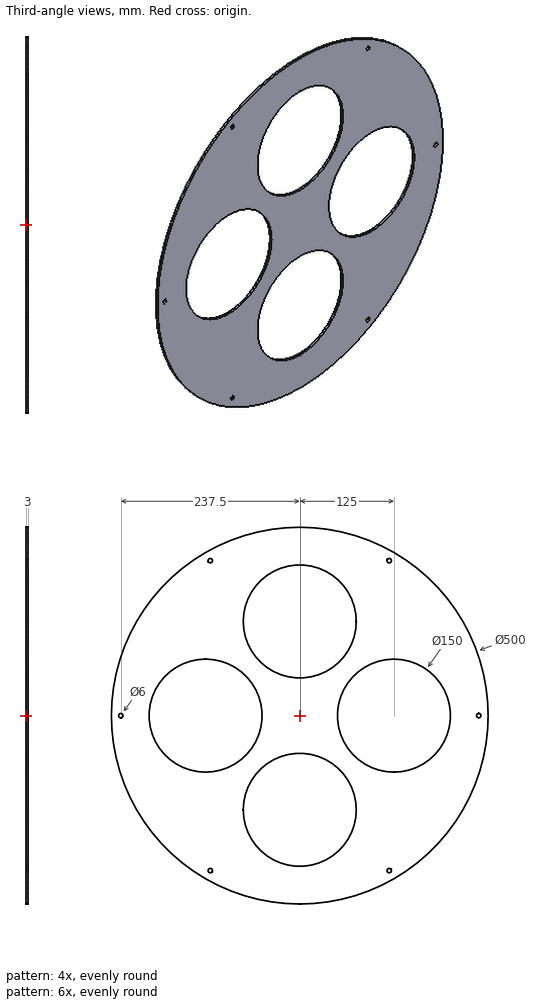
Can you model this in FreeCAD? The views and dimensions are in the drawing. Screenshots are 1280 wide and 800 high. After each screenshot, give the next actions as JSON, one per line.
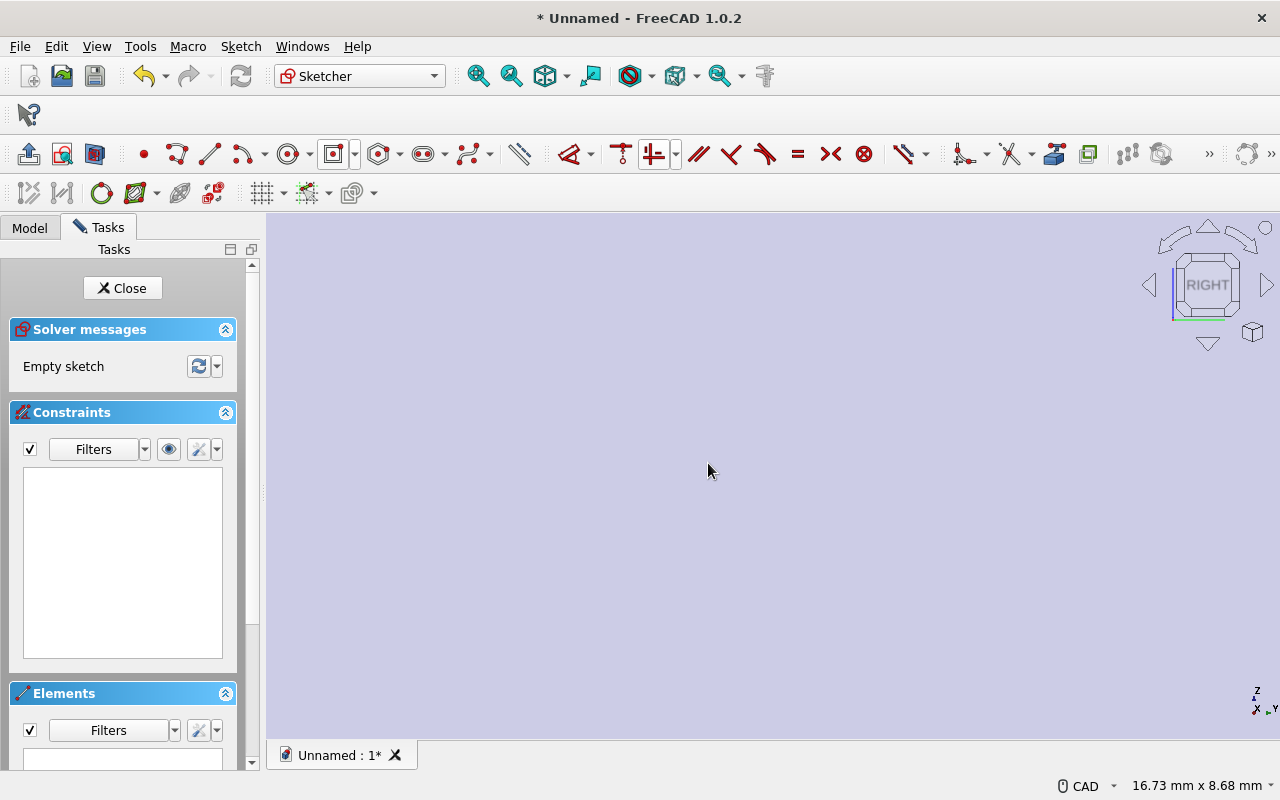
{"action": "left_click", "coordinate": [288, 154]}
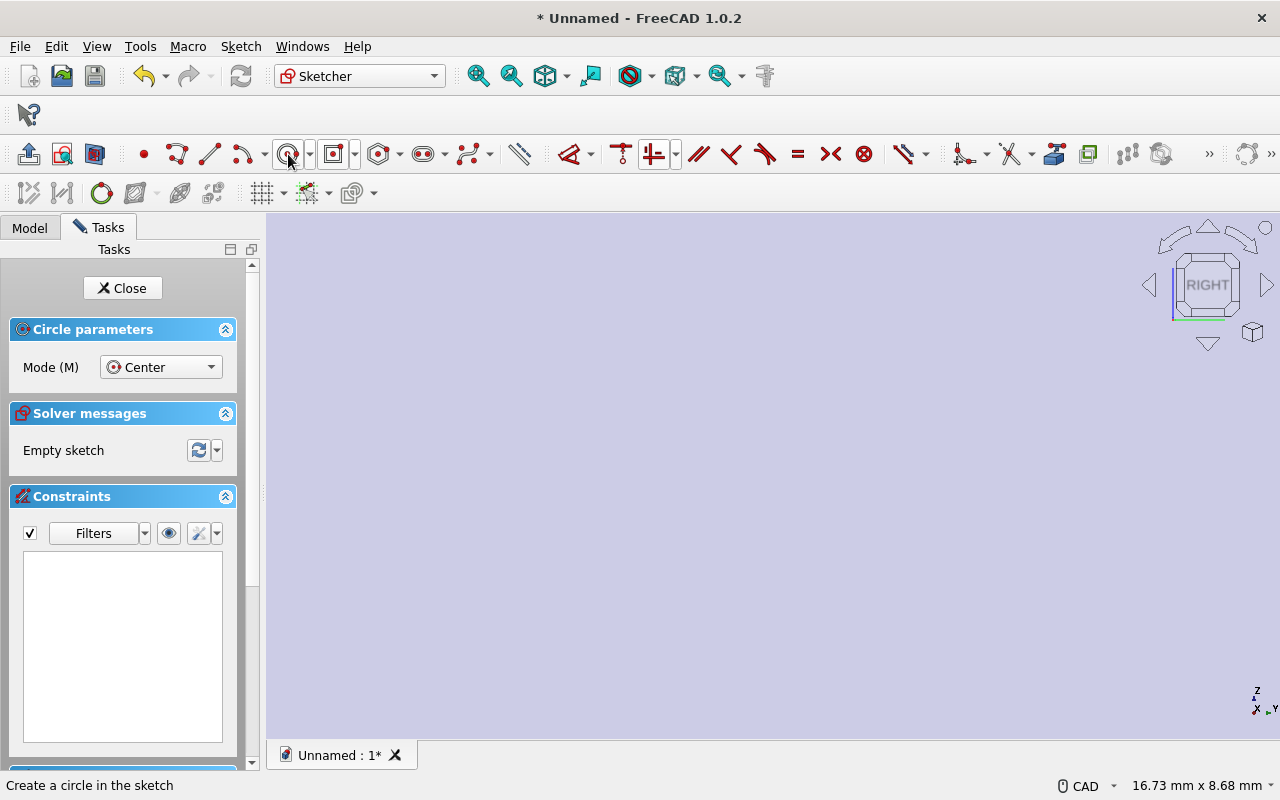
{"action": "left_click", "coordinate": [702, 475]}
{"action": "mouse_move", "coordinate": [830, 347]}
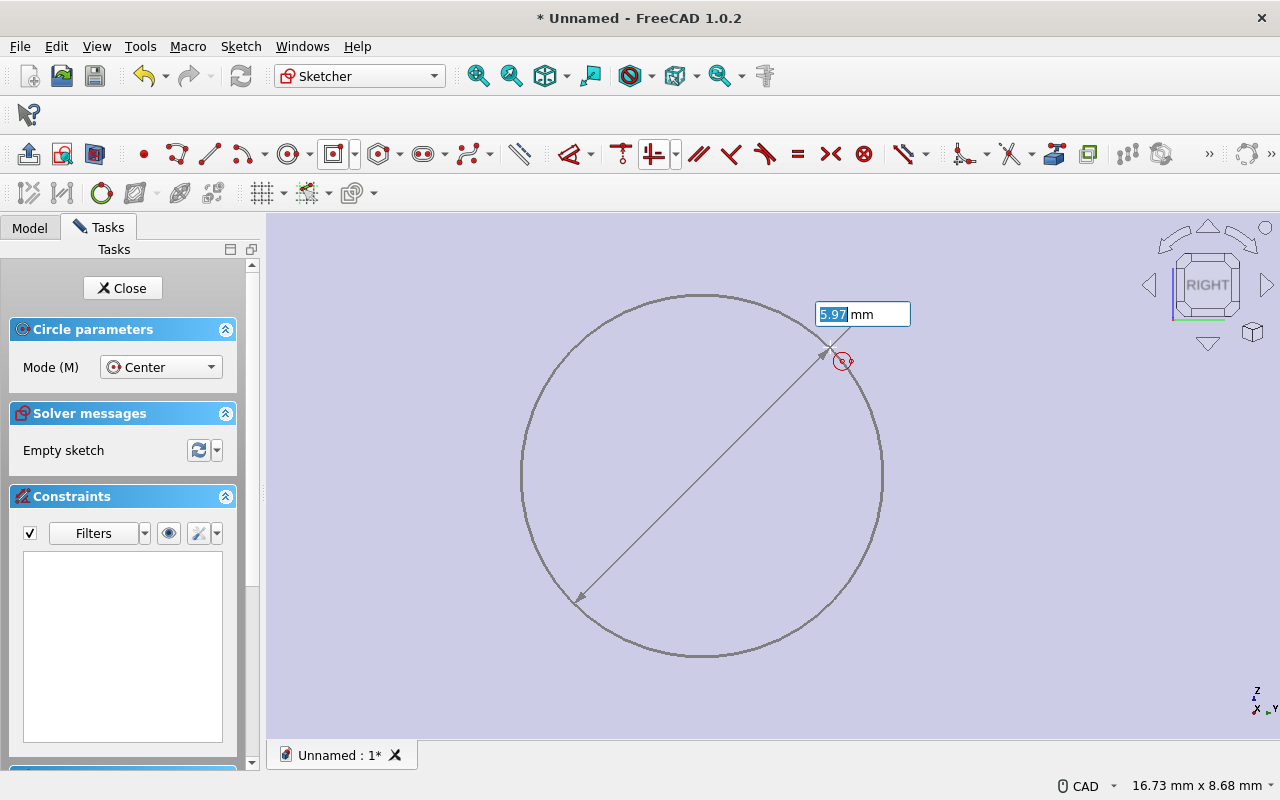
{"action": "type", "text": "6"}
{"action": "key", "text": "Return"}
{"action": "key", "text": "Escape"}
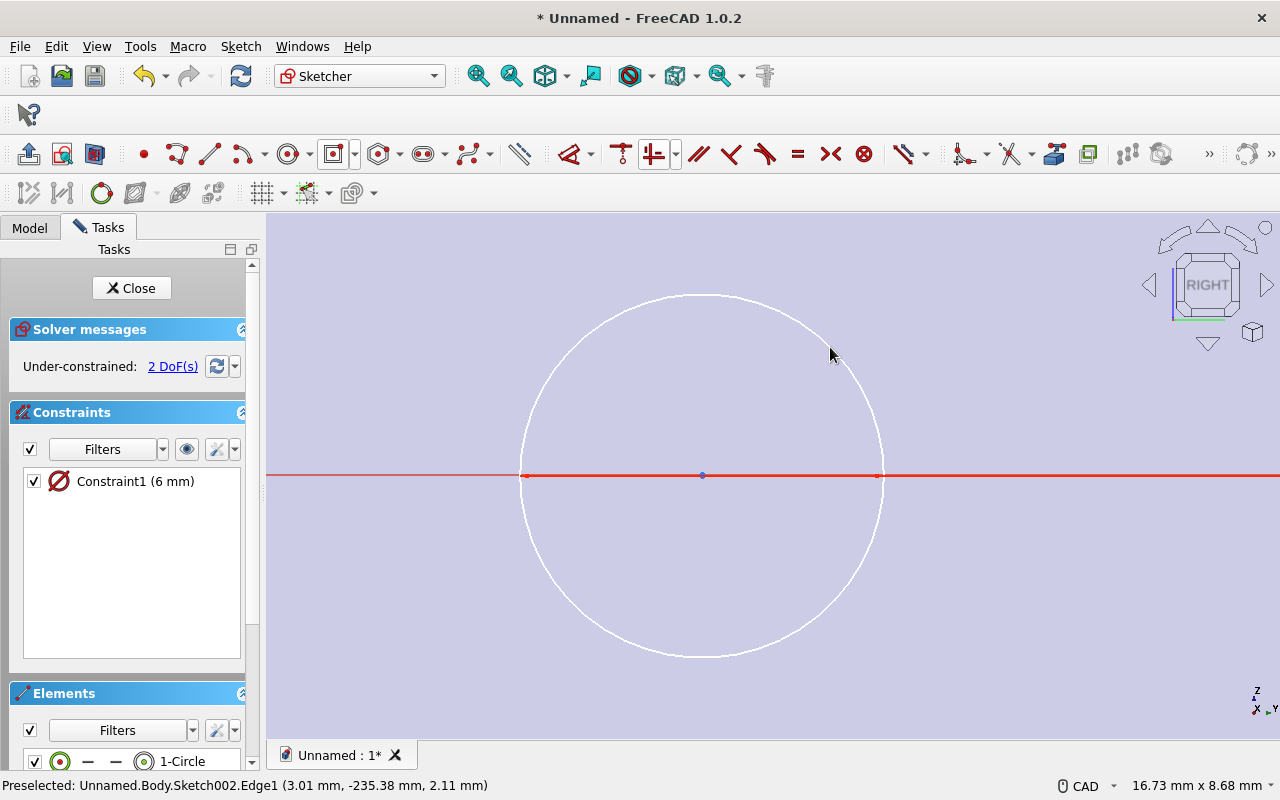
{"action": "left_click", "coordinate": [702, 476]}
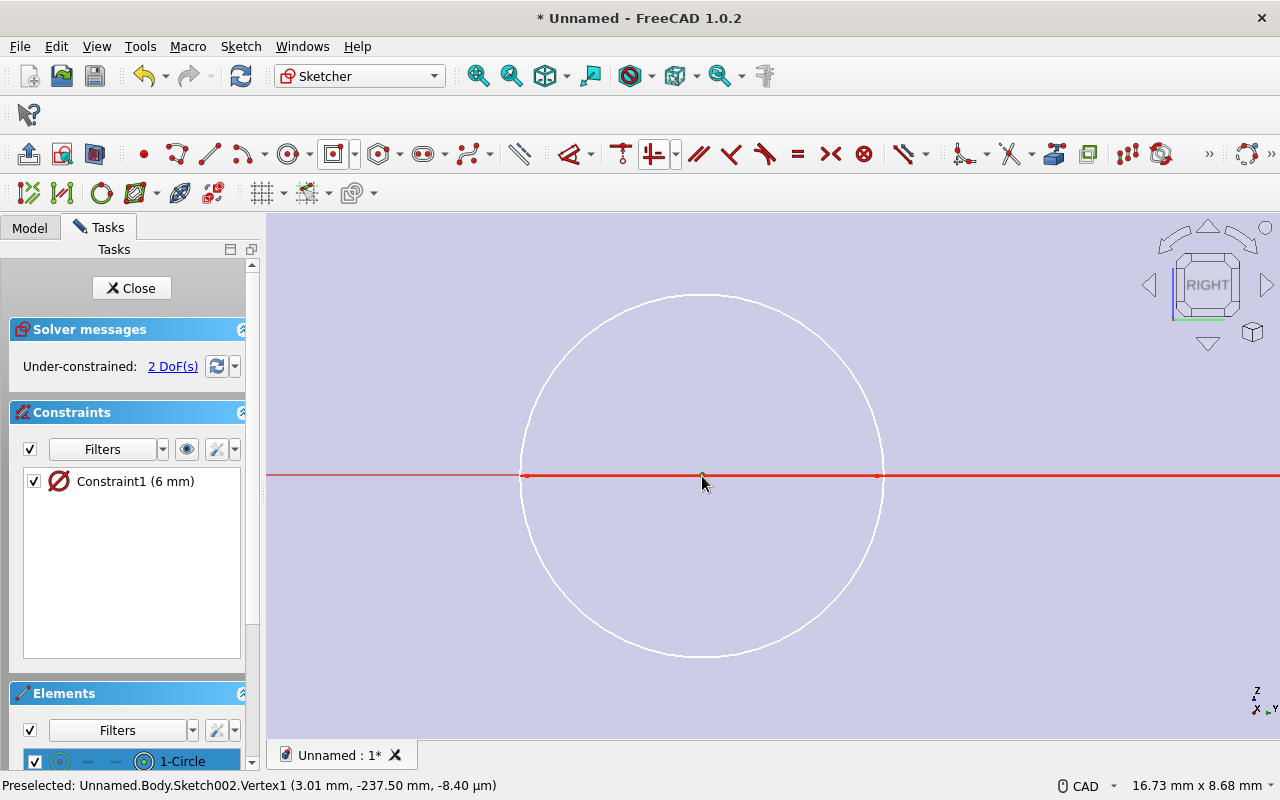
{"action": "left_click", "coordinate": [353, 475]}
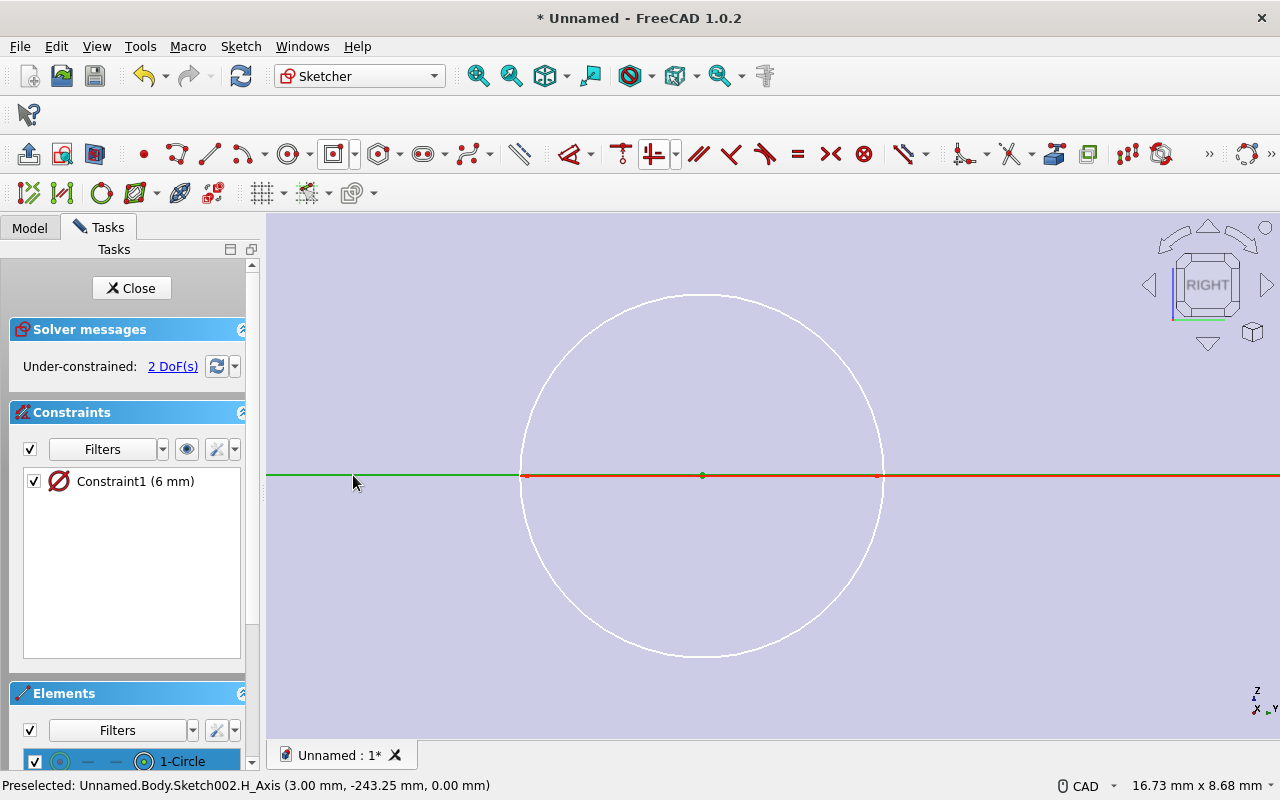
{"action": "left_click", "coordinate": [621, 154]}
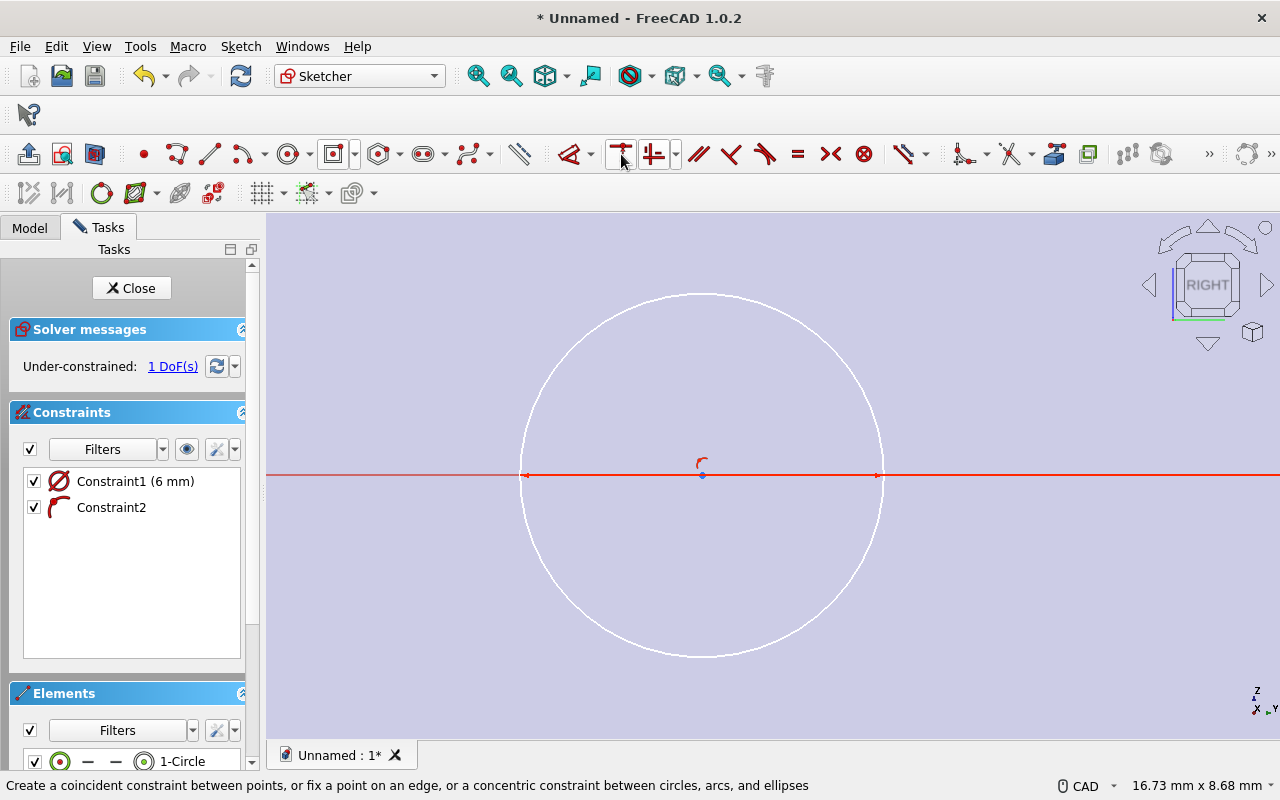
{"action": "left_click", "coordinate": [568, 154]}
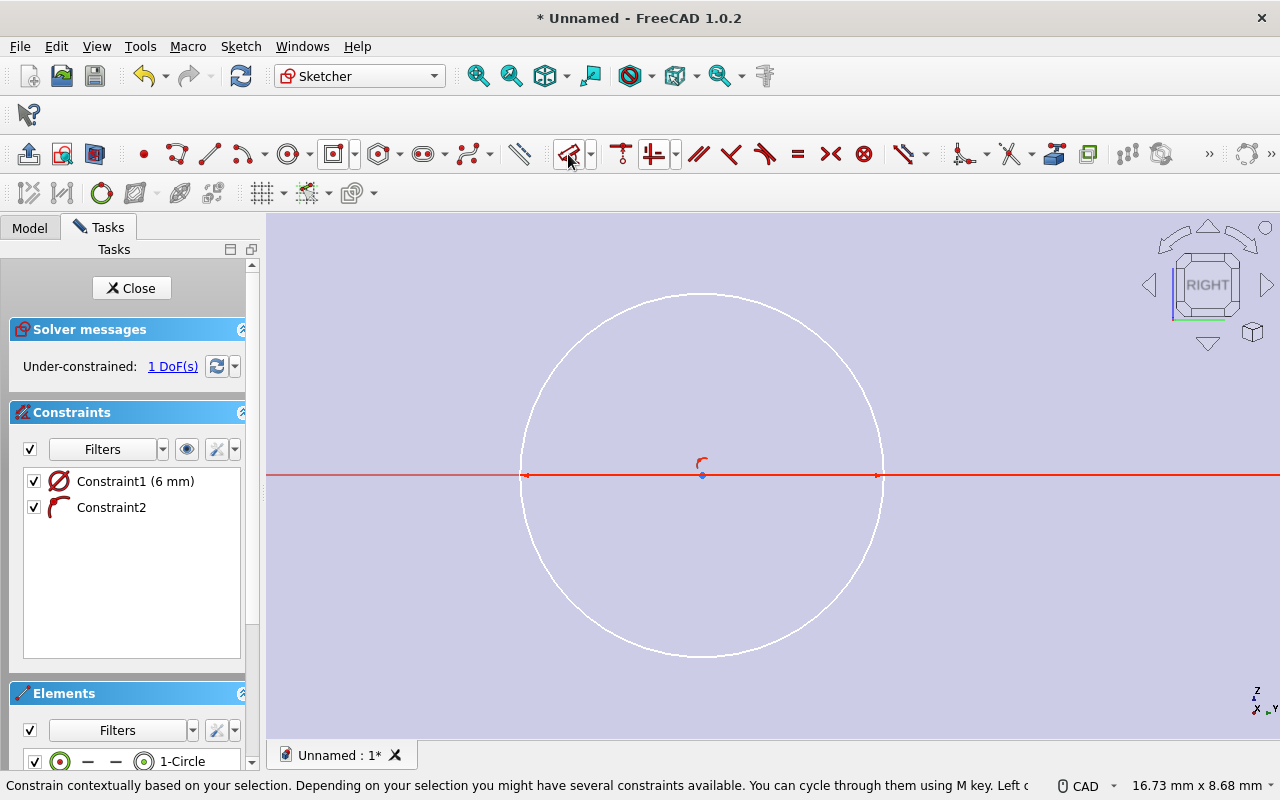
{"action": "left_click", "coordinate": [702, 475]}
{"action": "left_click", "coordinate": [909, 509]}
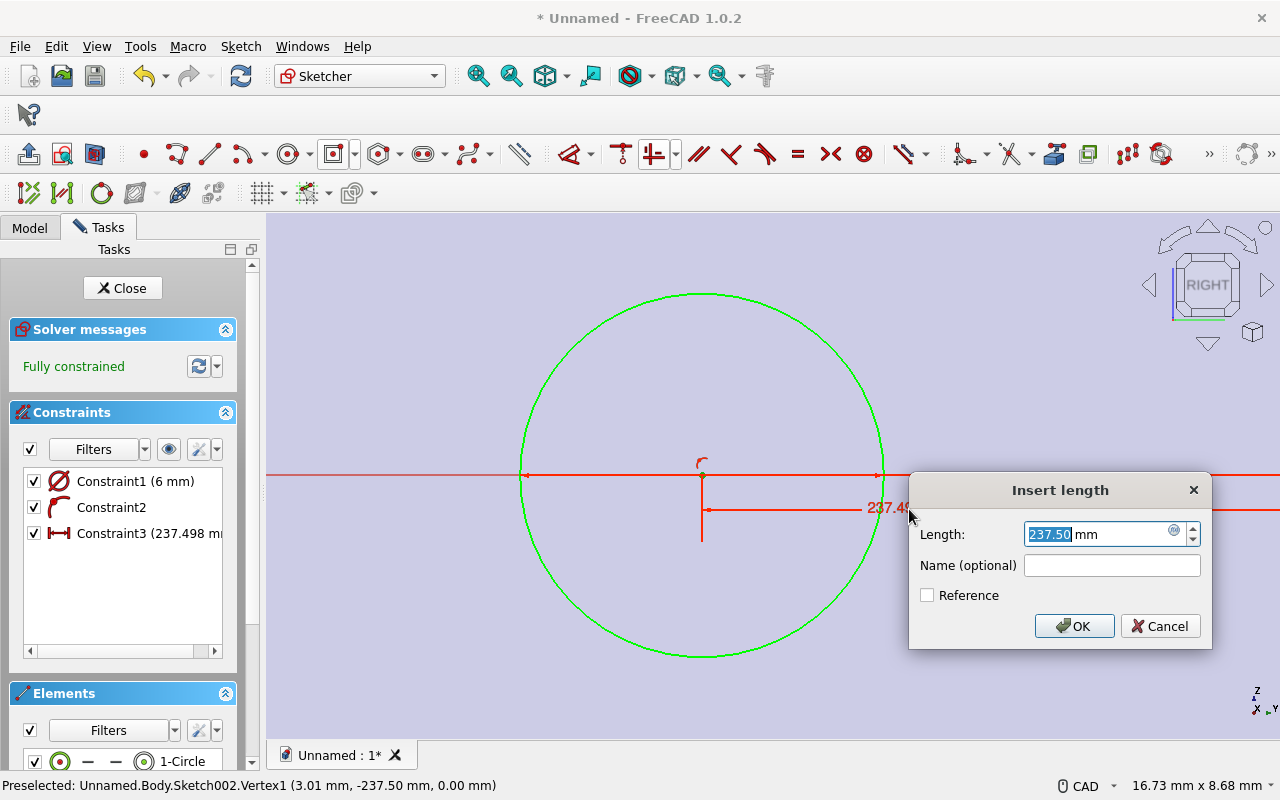
{"action": "type", "text": "237.5"}
{"action": "key", "text": "Return"}
{"action": "key", "text": "Escape"}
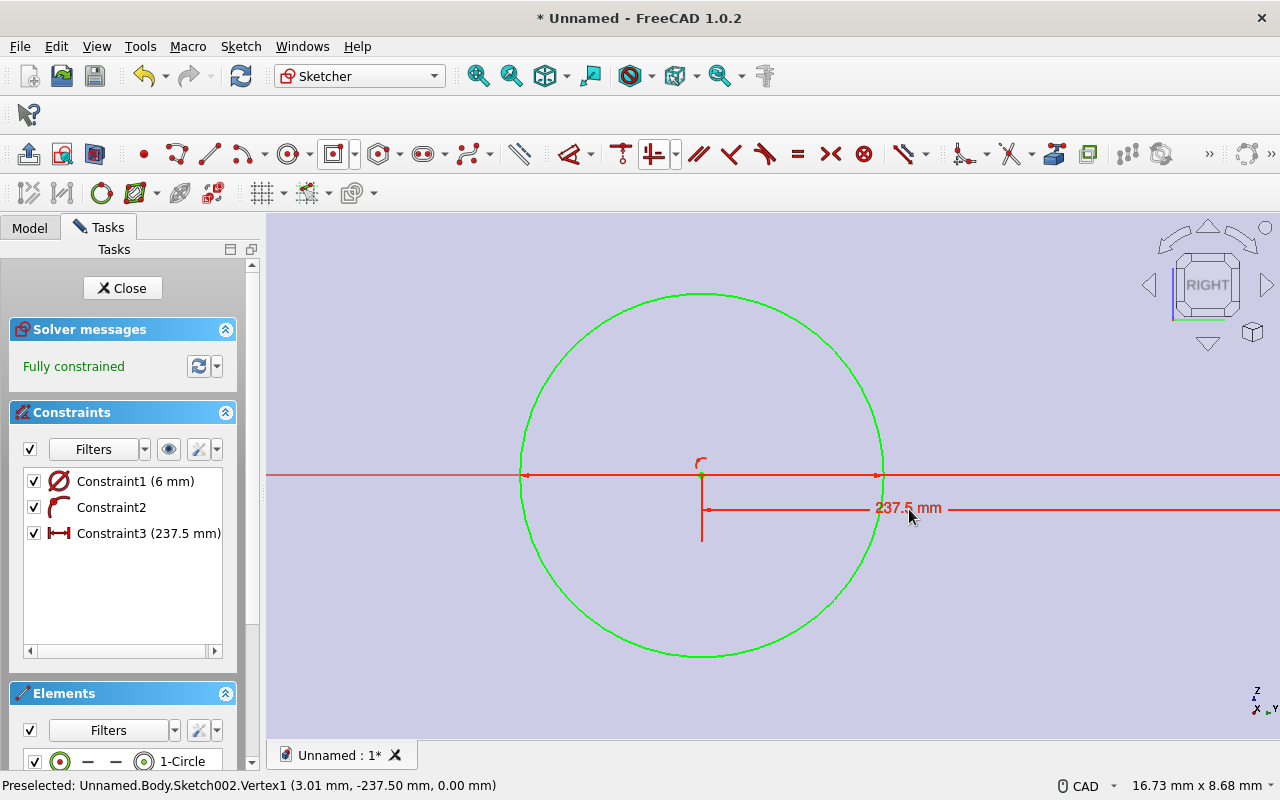
{"action": "left_click", "coordinate": [123, 288]}